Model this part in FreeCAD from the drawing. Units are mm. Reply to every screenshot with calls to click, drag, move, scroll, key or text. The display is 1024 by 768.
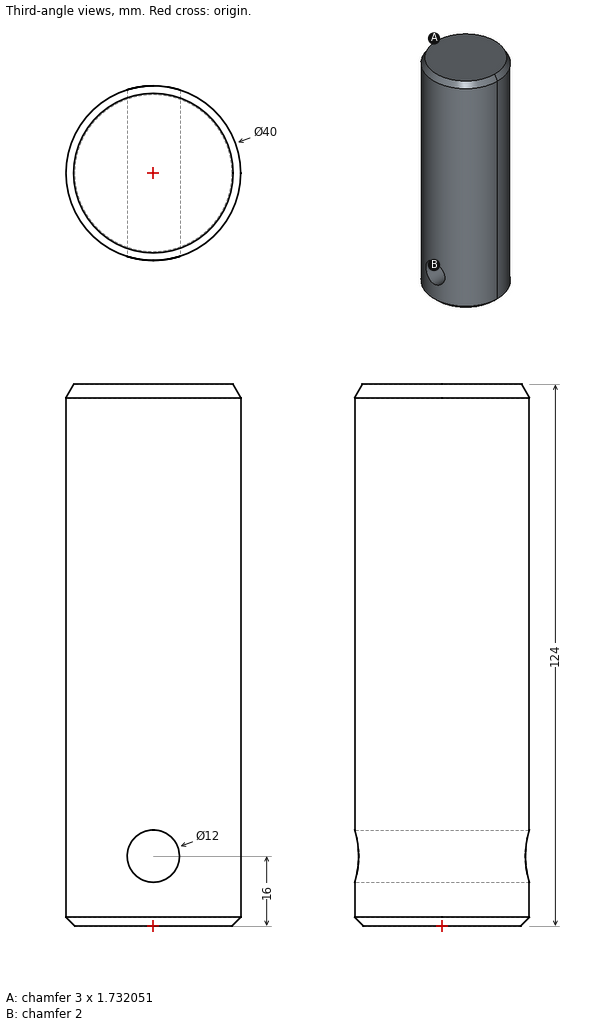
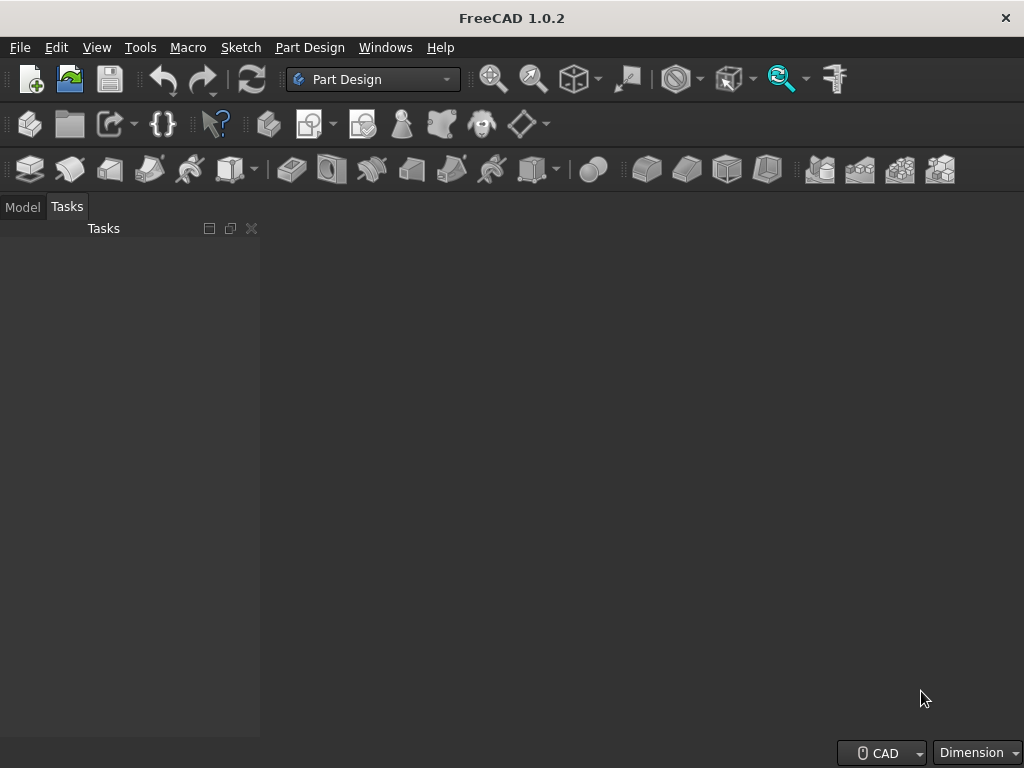
click(30, 80)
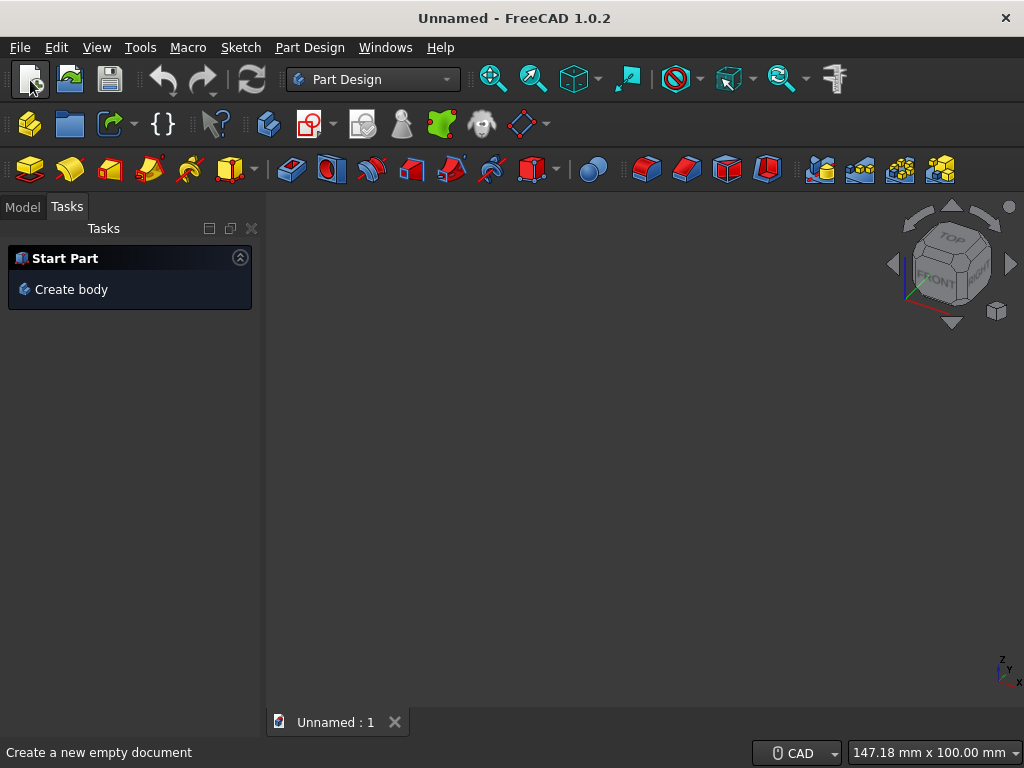
click(310, 124)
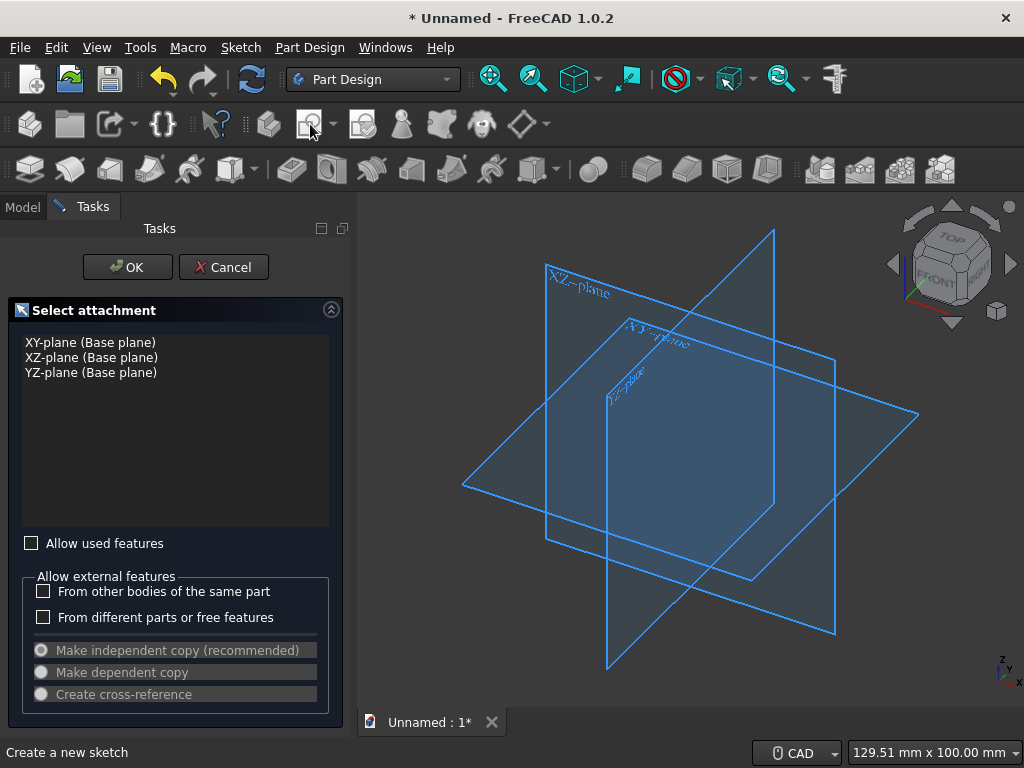
click(82, 342)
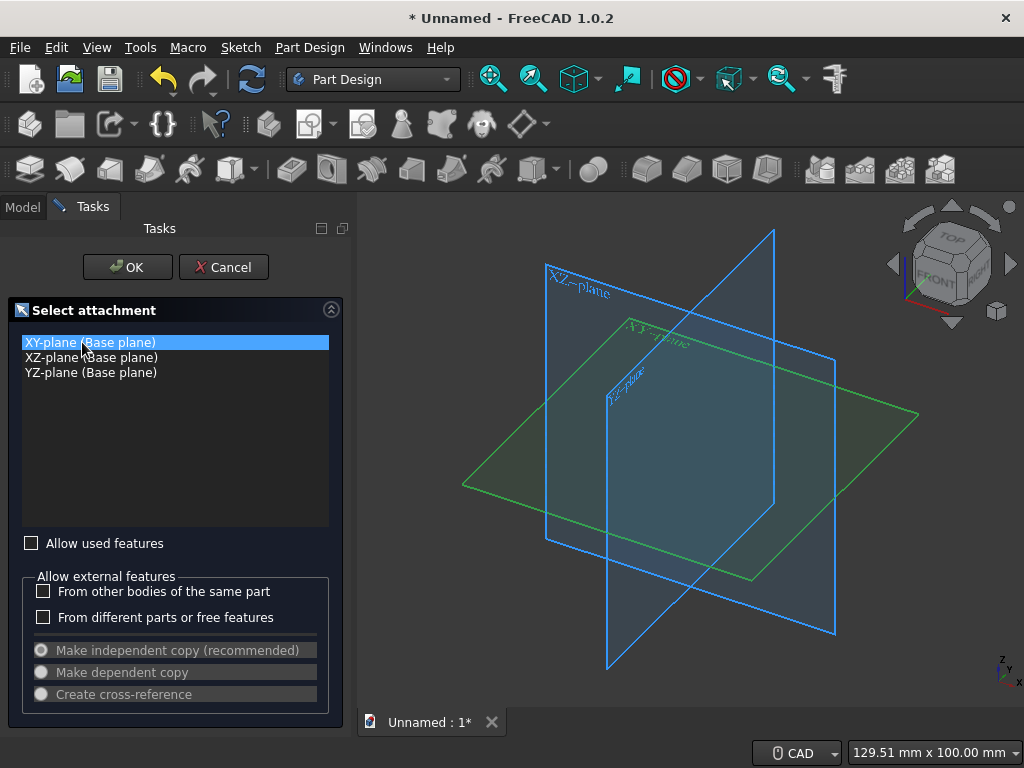
click(128, 267)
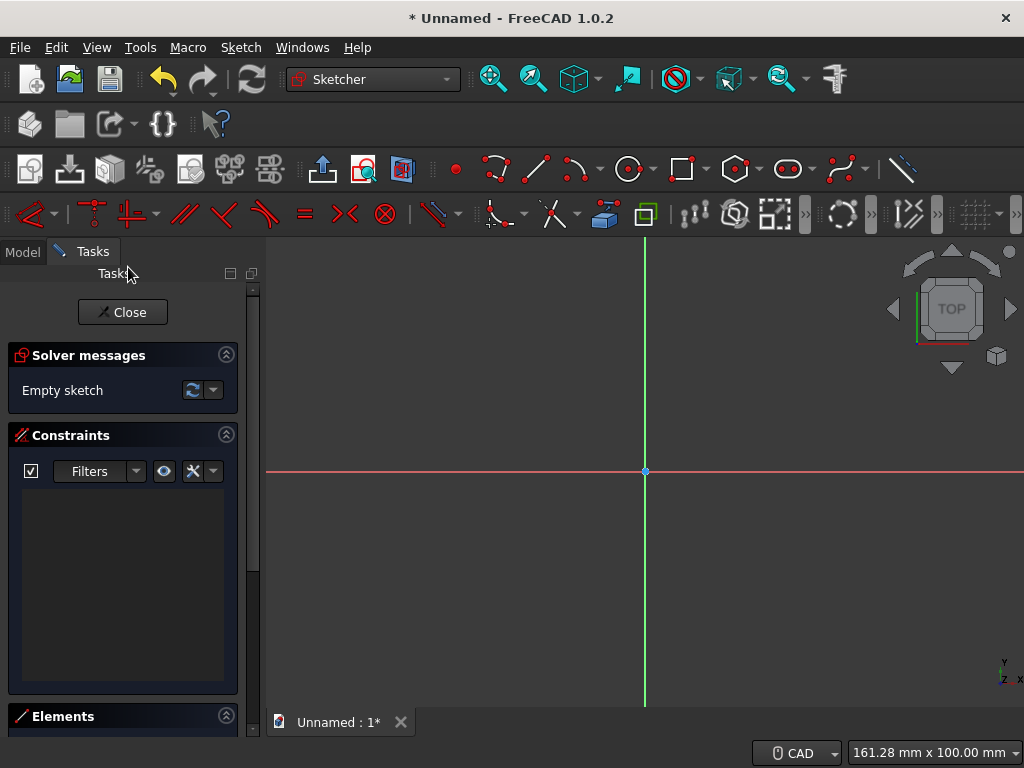
scroll(784, 472, up, 2)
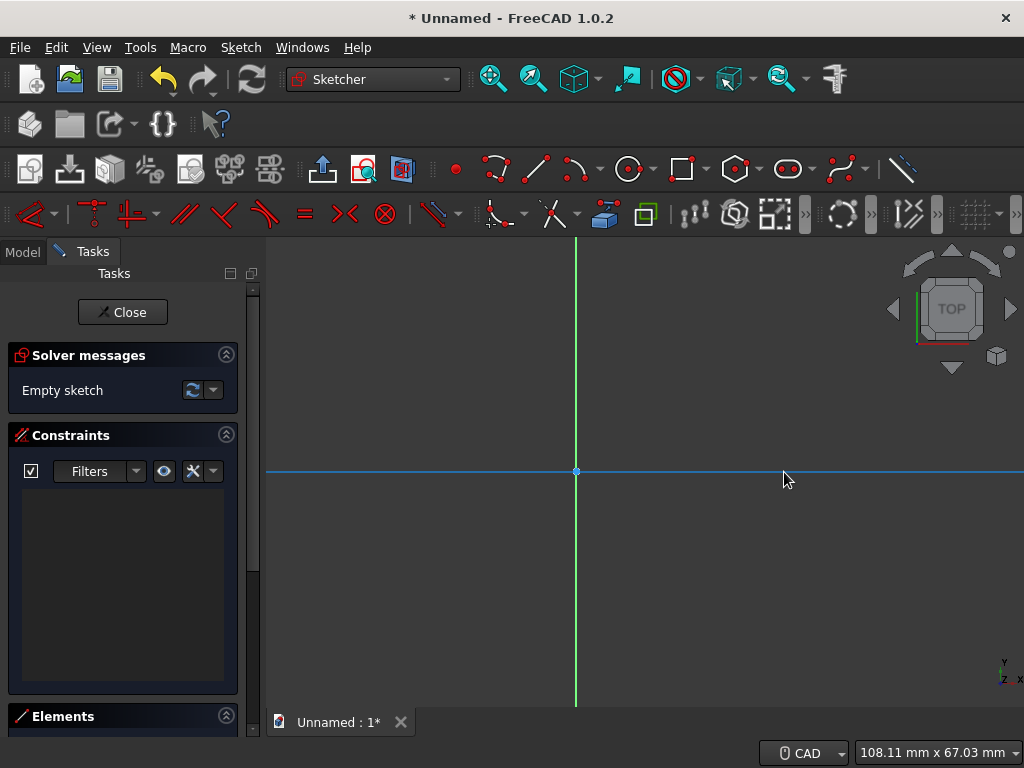
key(g)
key(c)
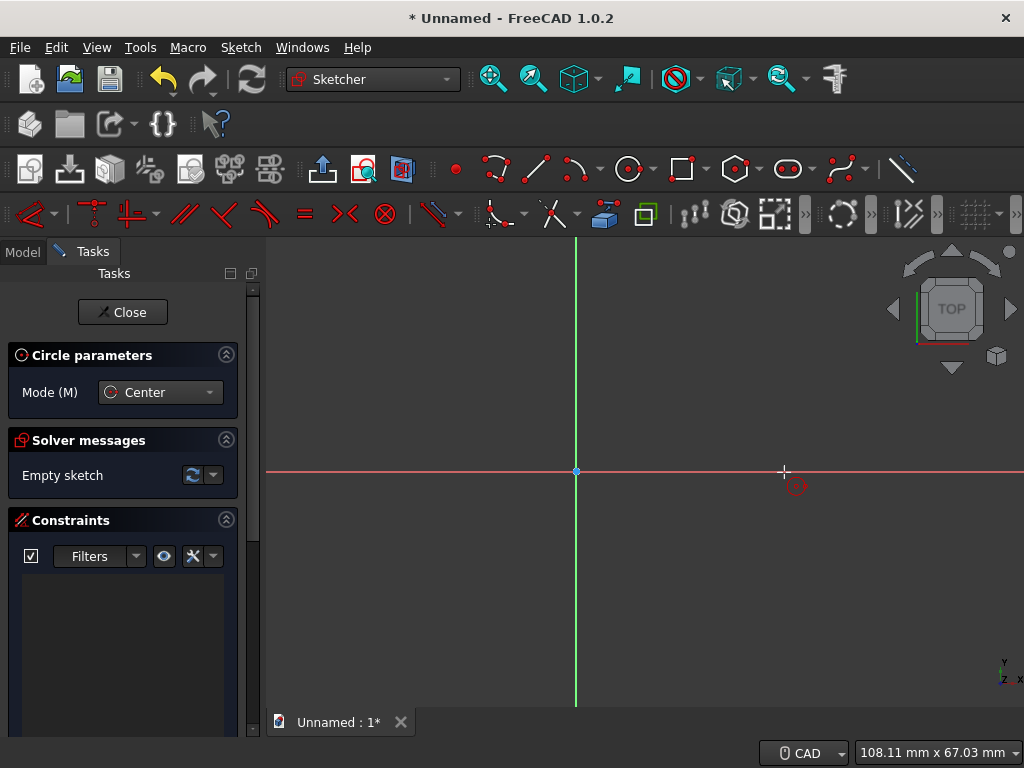
click(576, 472)
move(675, 373)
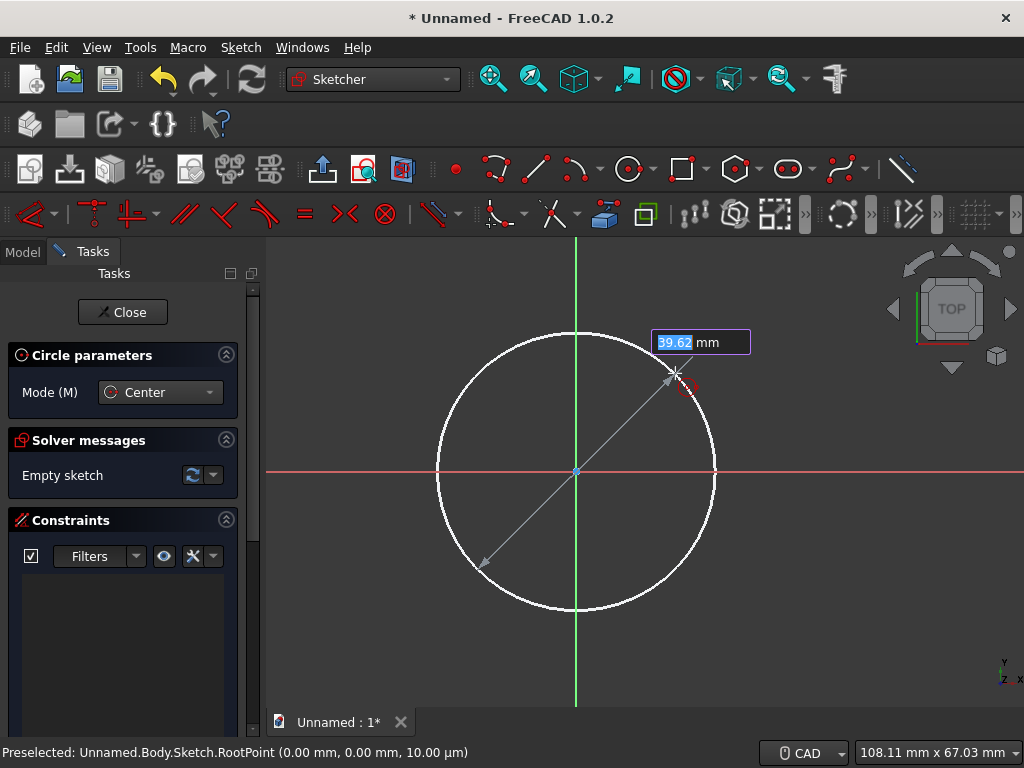
text(40)
key(Return)
key(Escape)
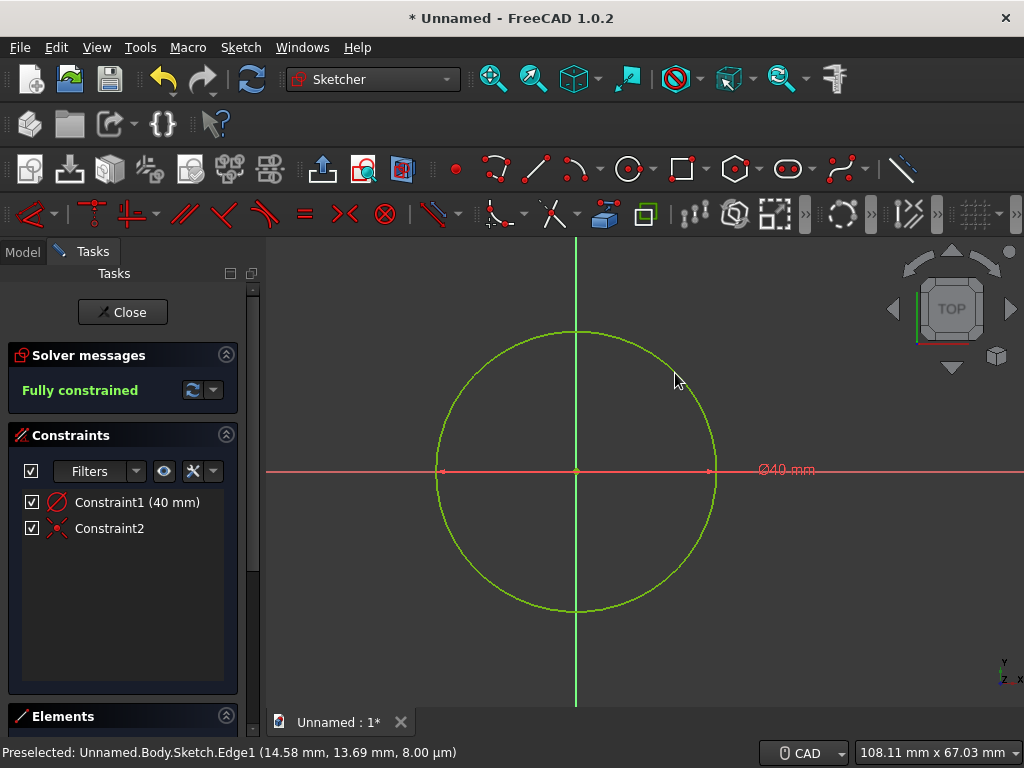
click(123, 312)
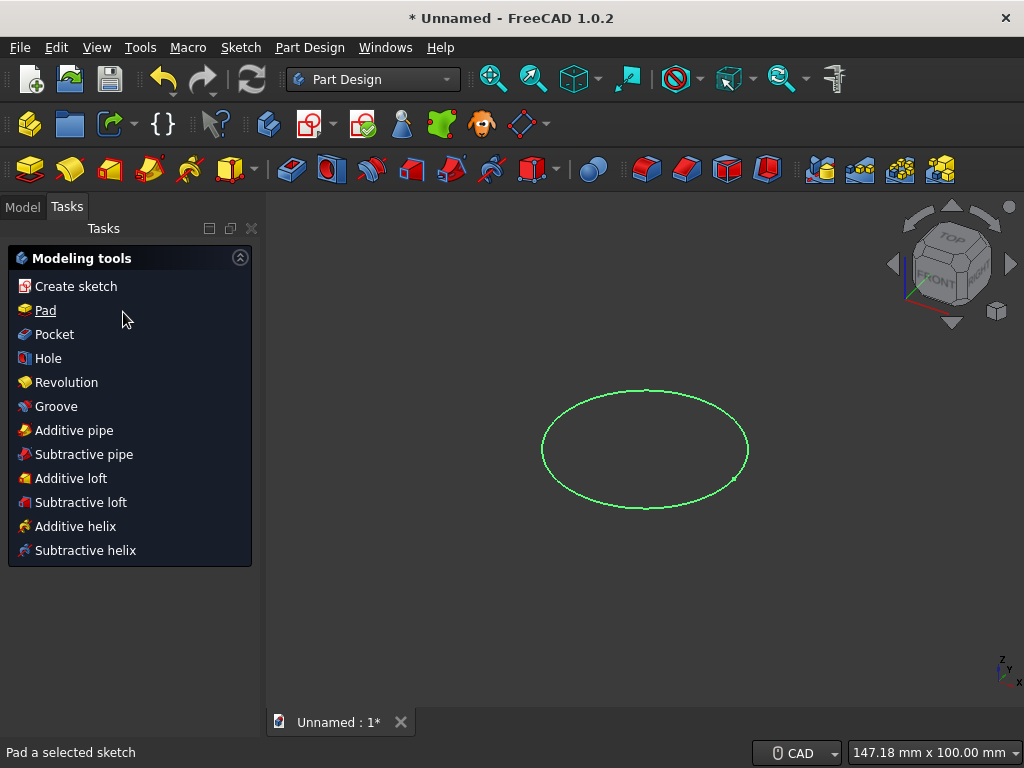
click(30, 170)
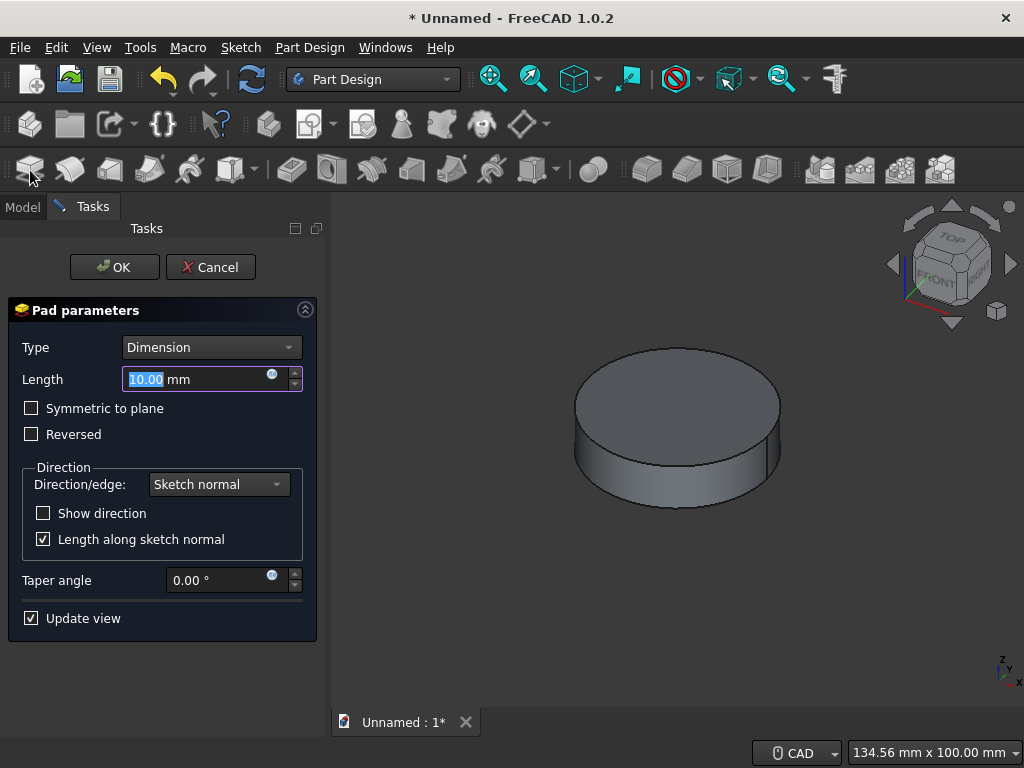
text(124)
key(Tab)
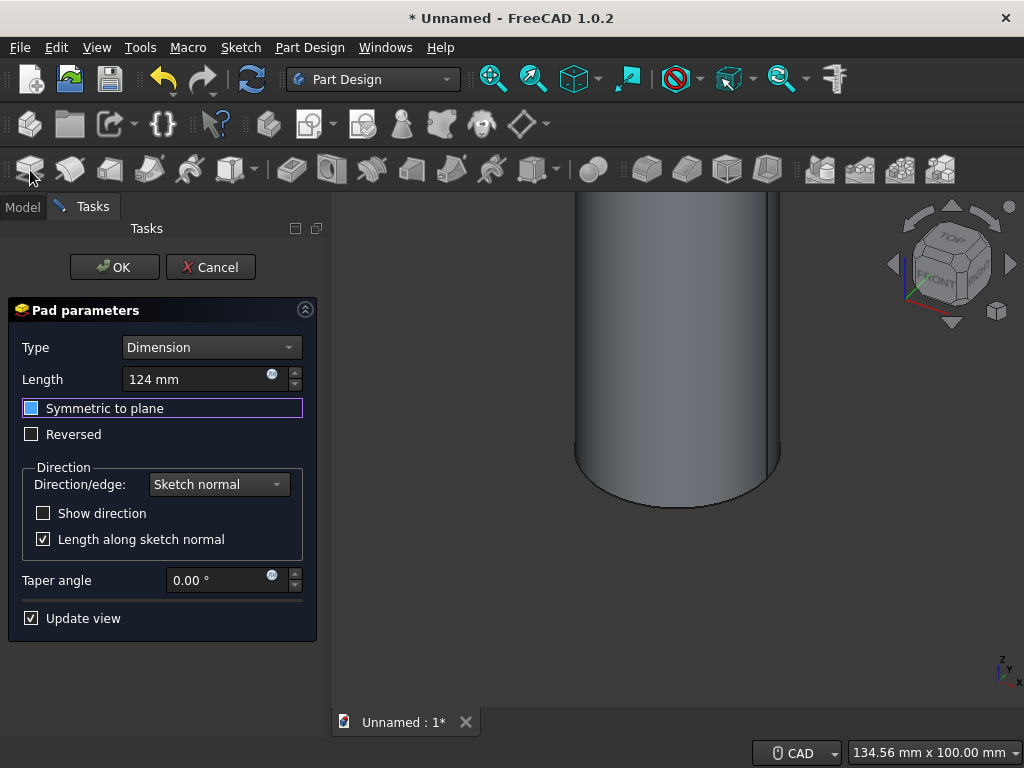
click(115, 267)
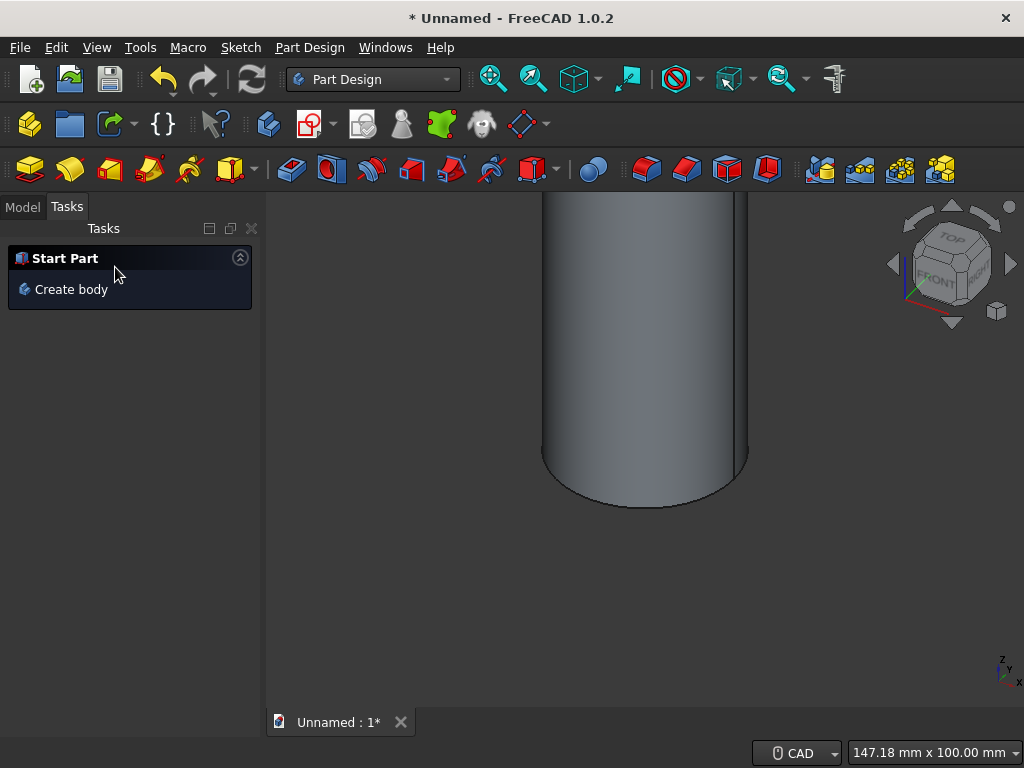
key(v)
key(f)